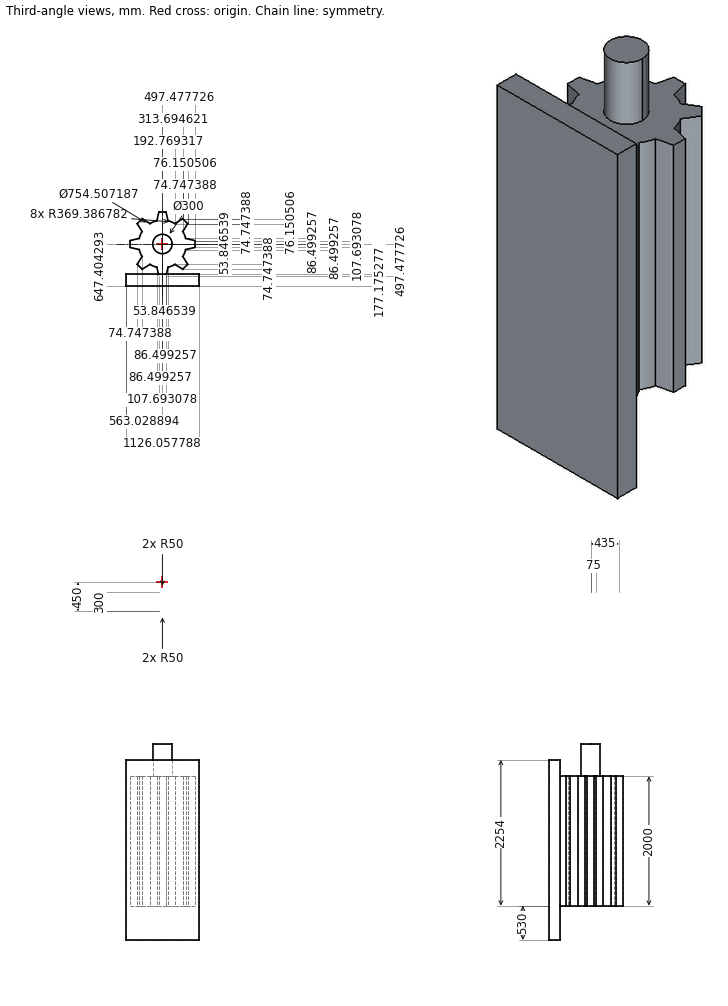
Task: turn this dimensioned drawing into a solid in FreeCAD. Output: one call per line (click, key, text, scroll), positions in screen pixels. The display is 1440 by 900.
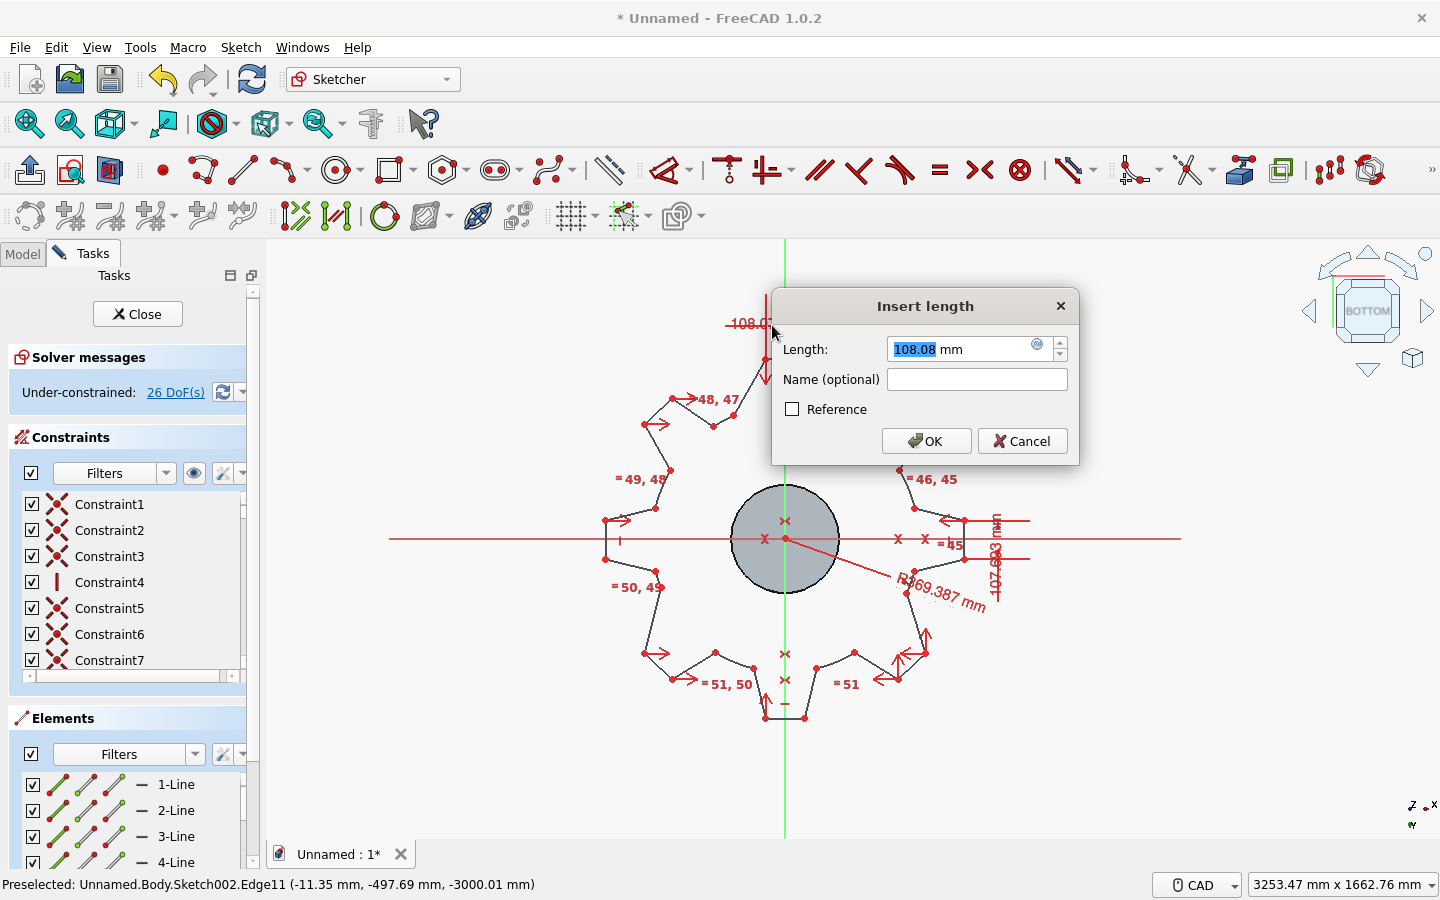
text(107.693078)
key(Return)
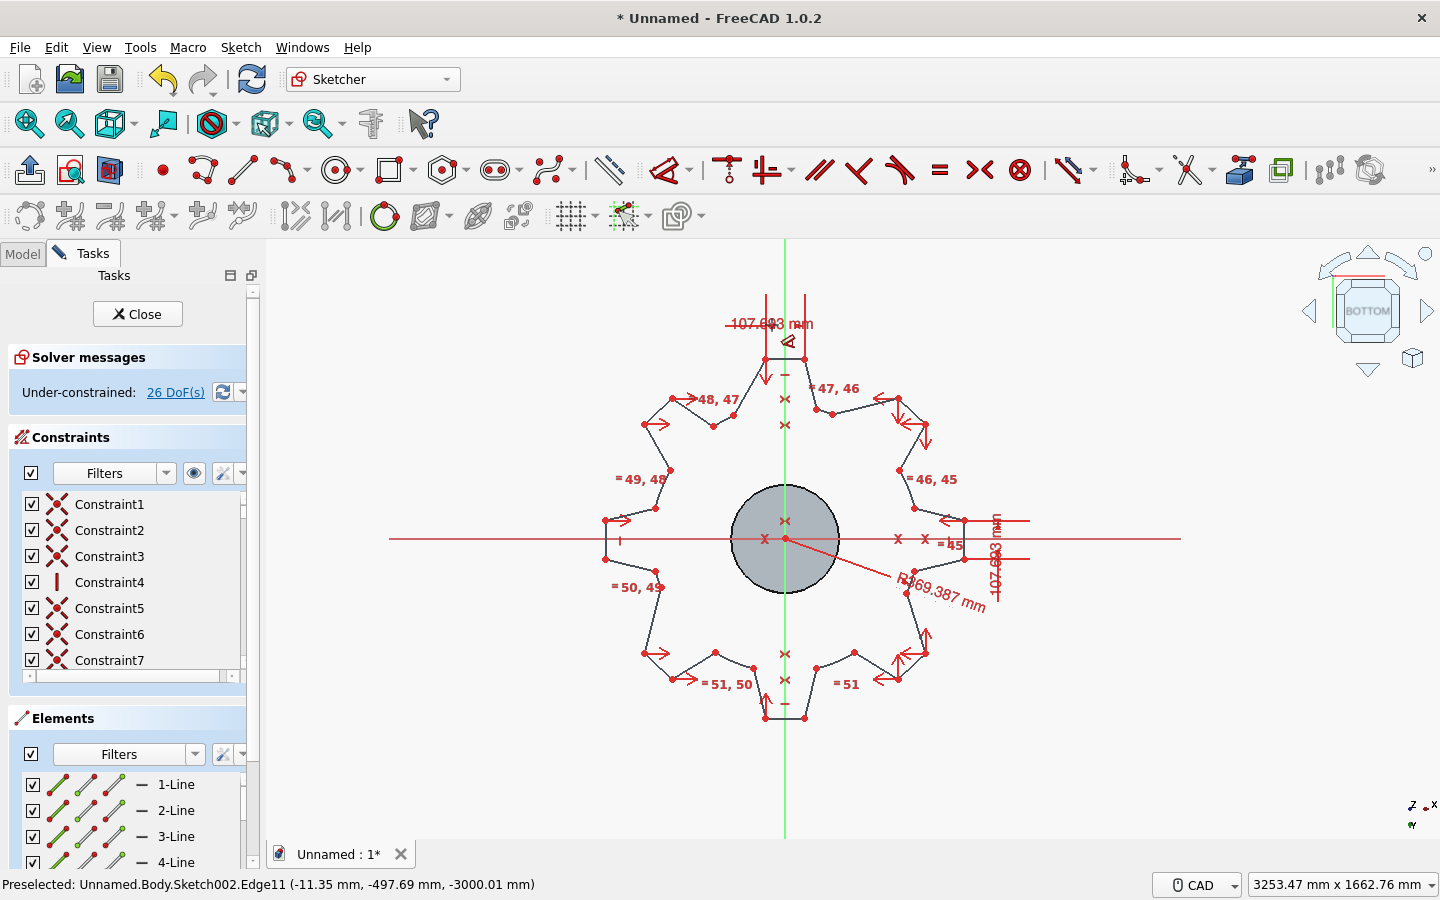
click(606, 536)
click(572, 554)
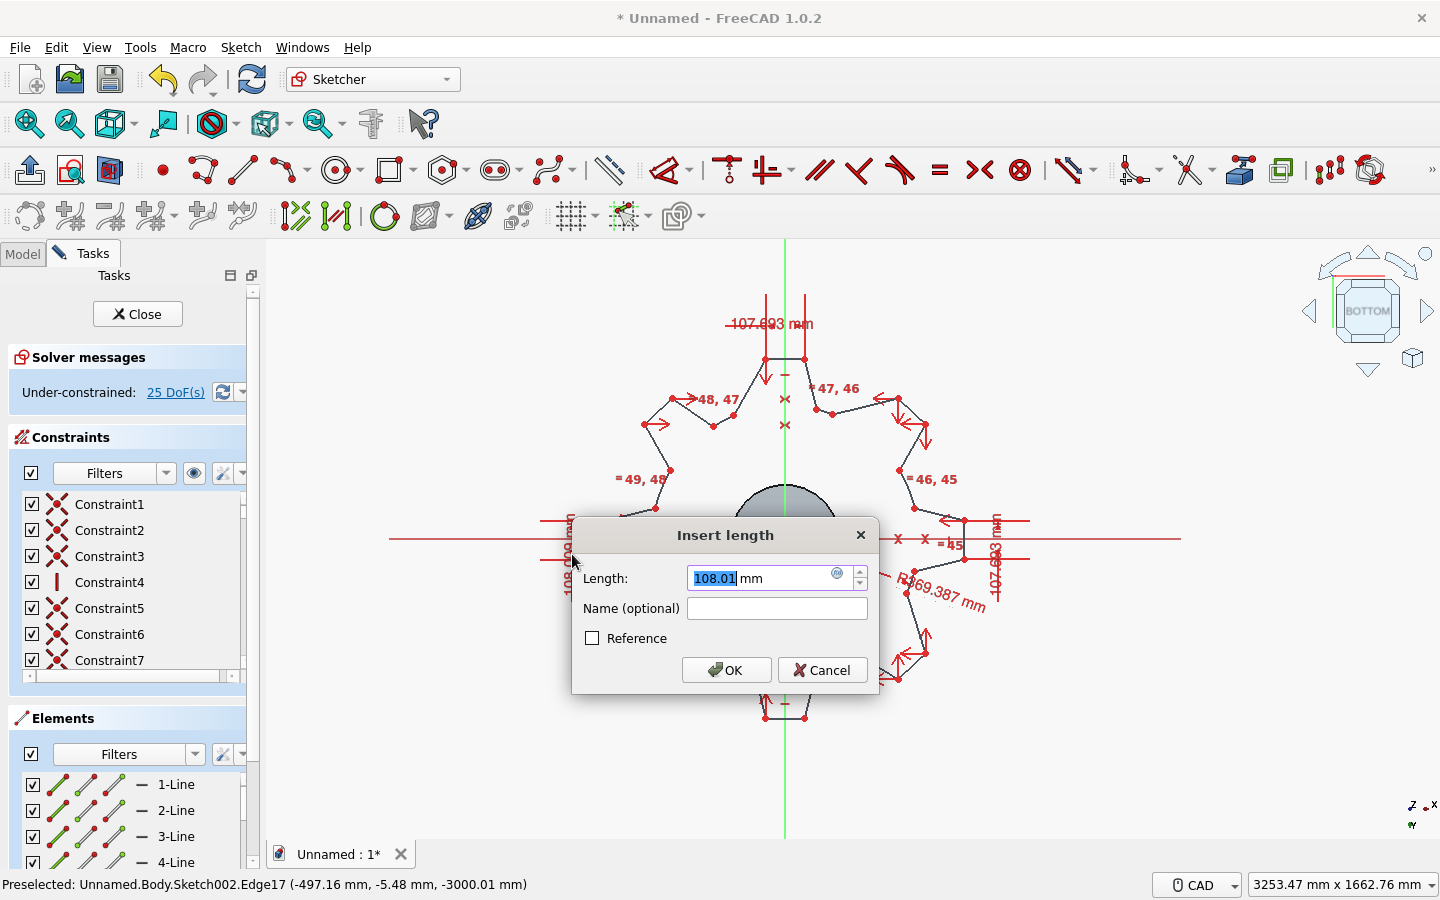
text(107.693078)
key(Return)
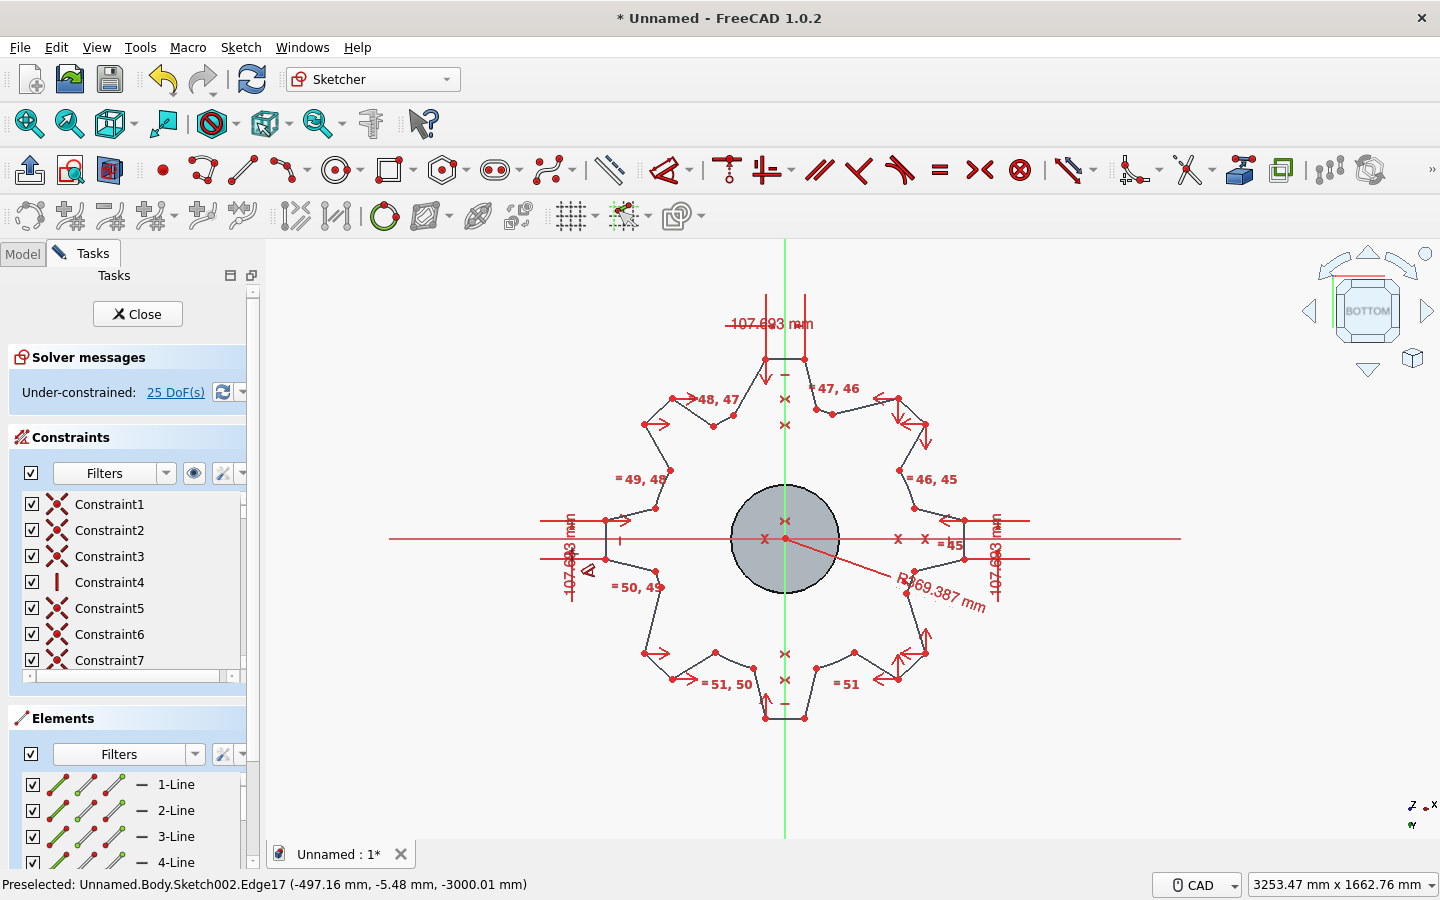
click(781, 719)
click(772, 753)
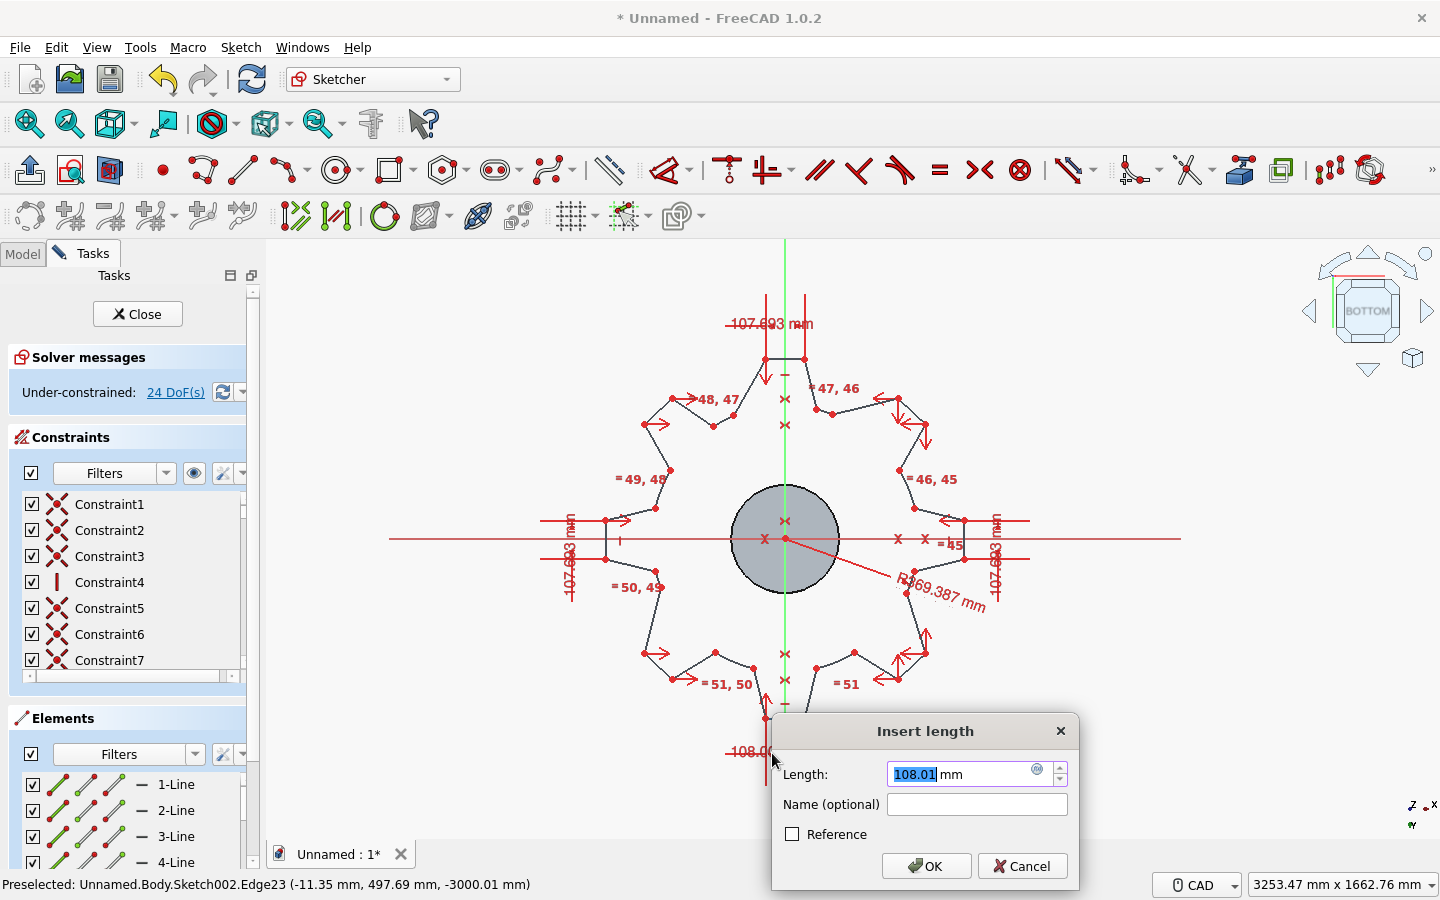
text(107.693078)
key(Return)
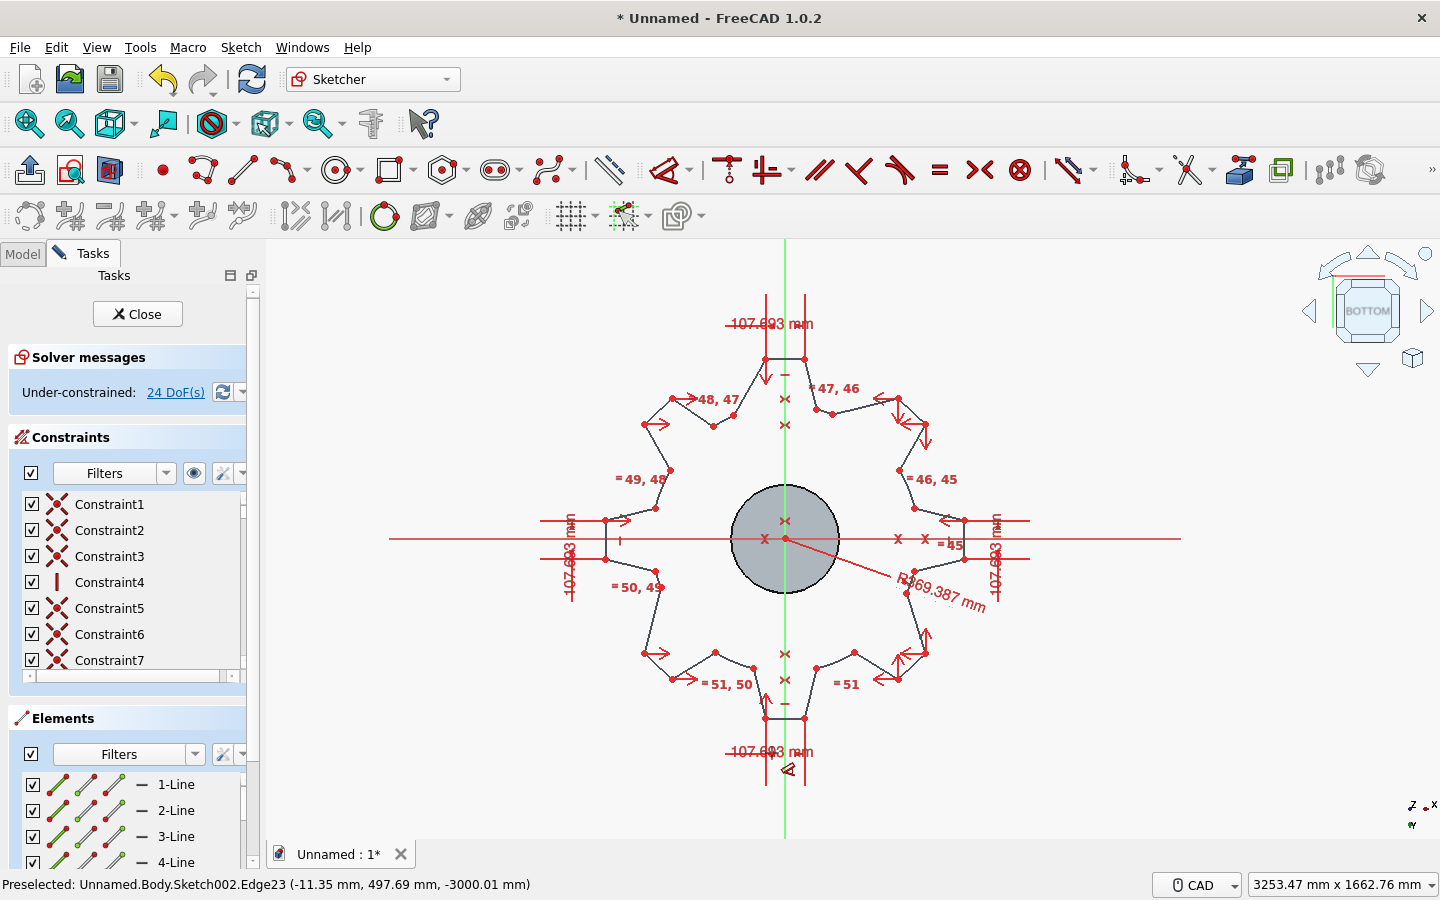
scroll(914, 572, up, 2)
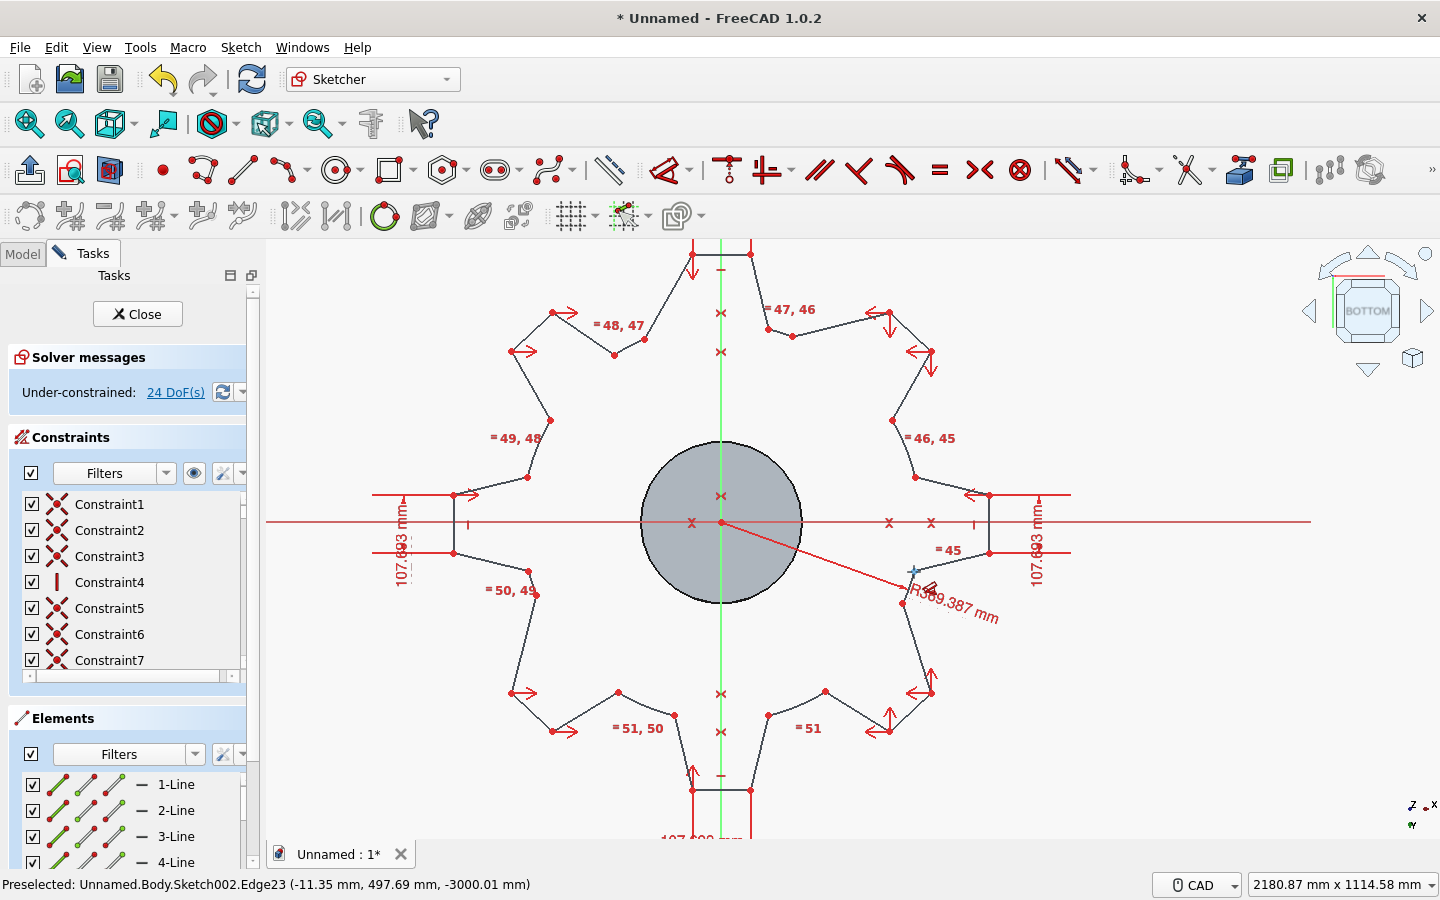
click(914, 571)
click(948, 547)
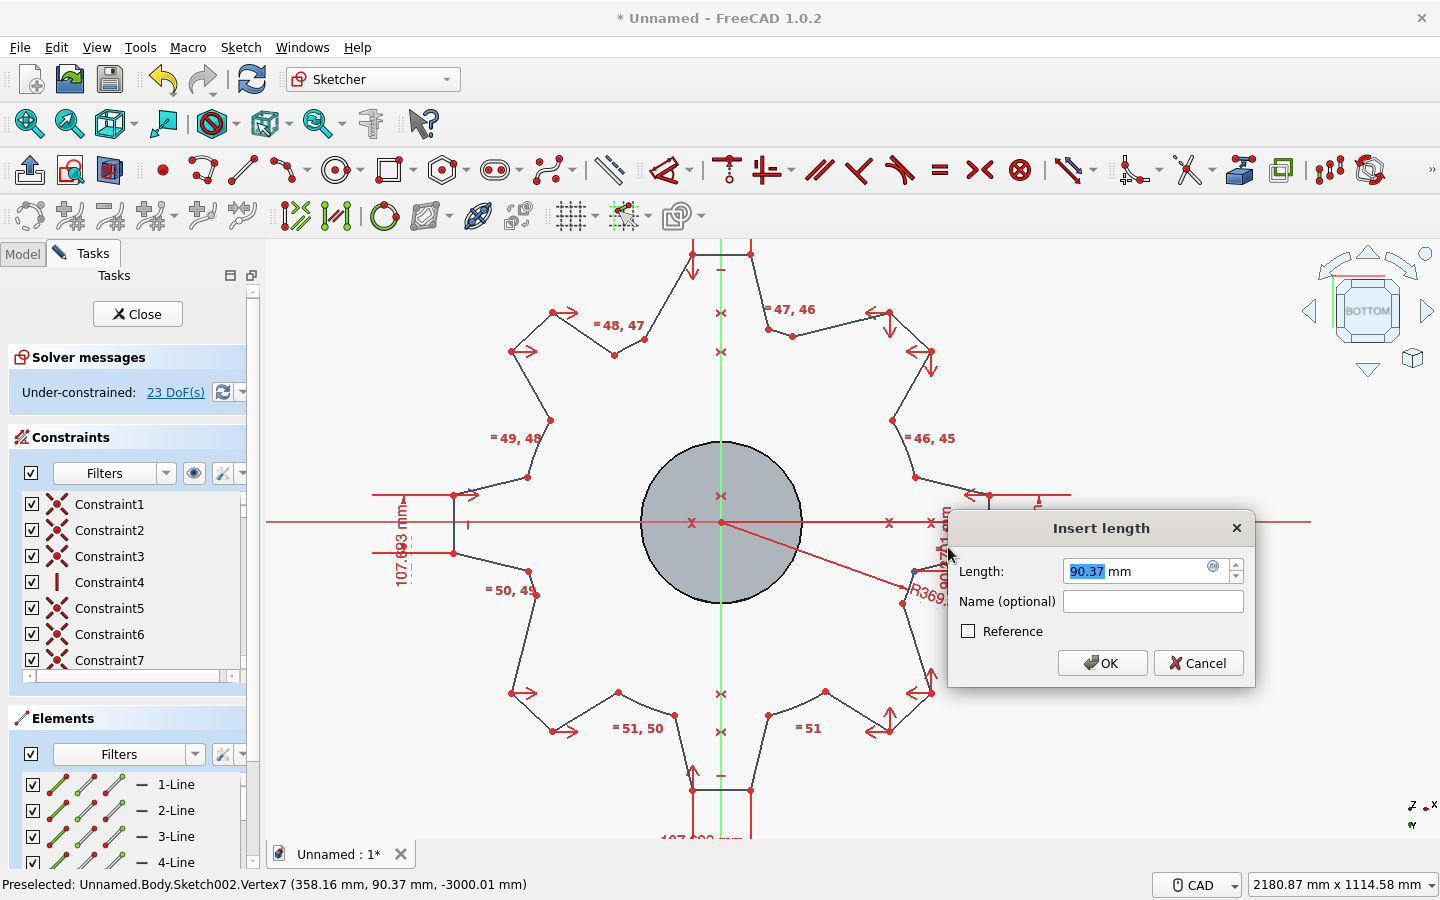
text(86.499257)
key(Return)